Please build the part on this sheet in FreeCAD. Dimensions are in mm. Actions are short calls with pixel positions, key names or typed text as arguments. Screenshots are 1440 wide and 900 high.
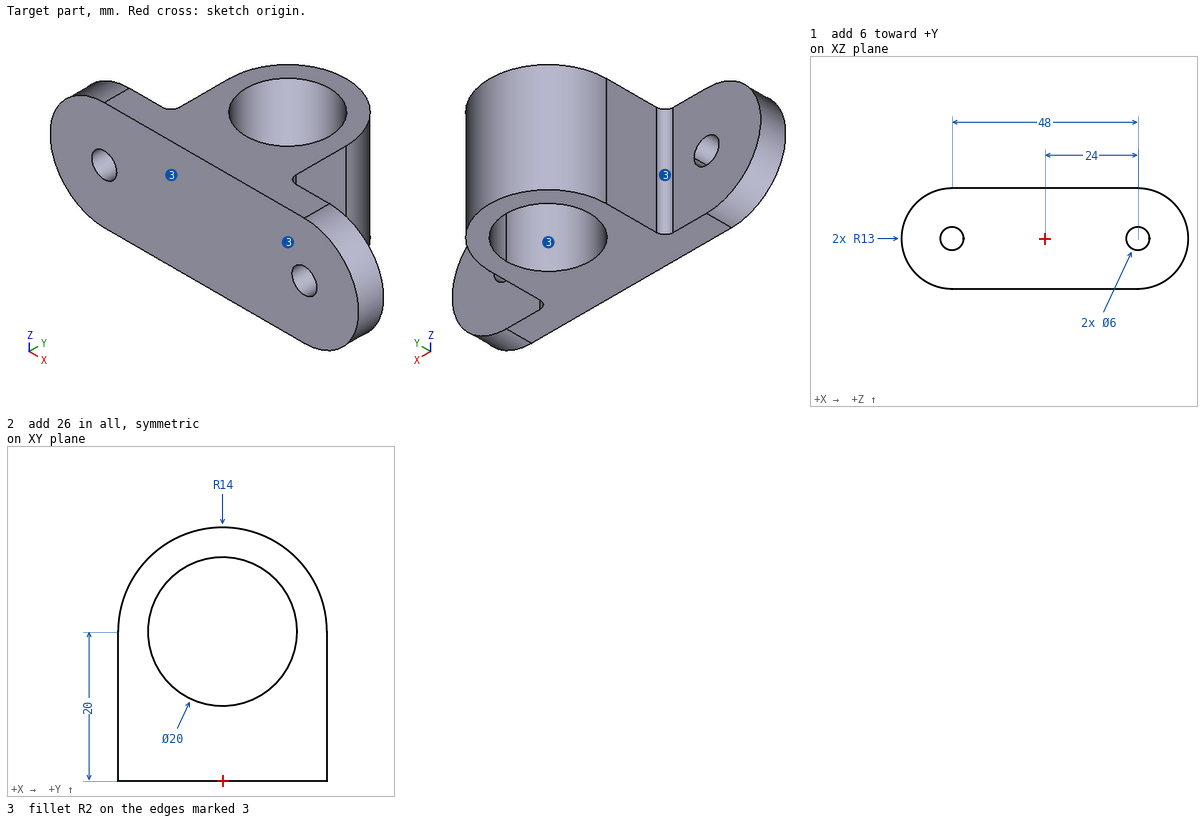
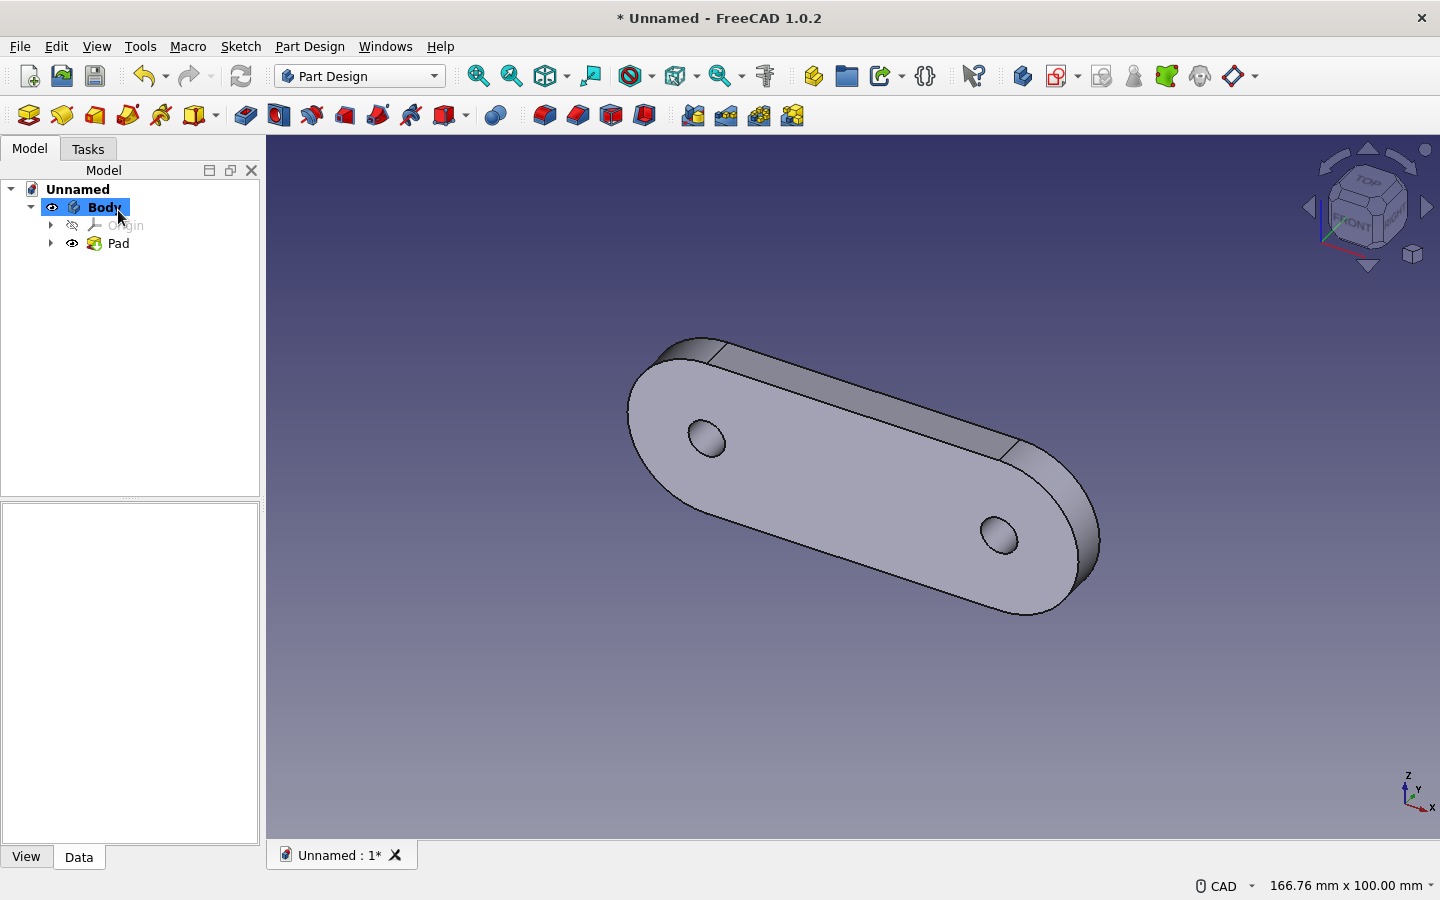
click(1056, 76)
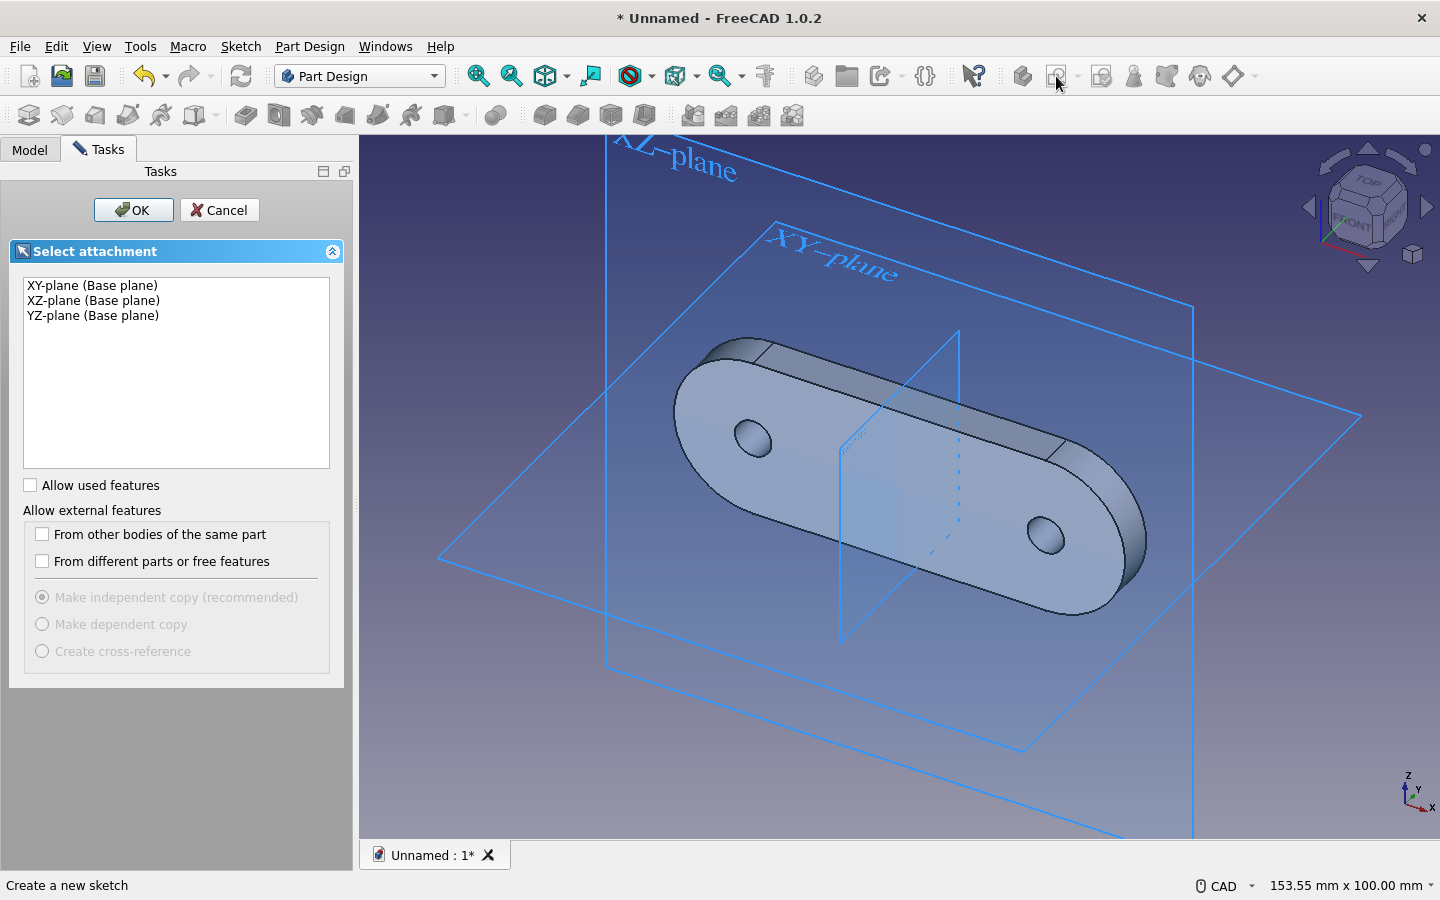
click(84, 286)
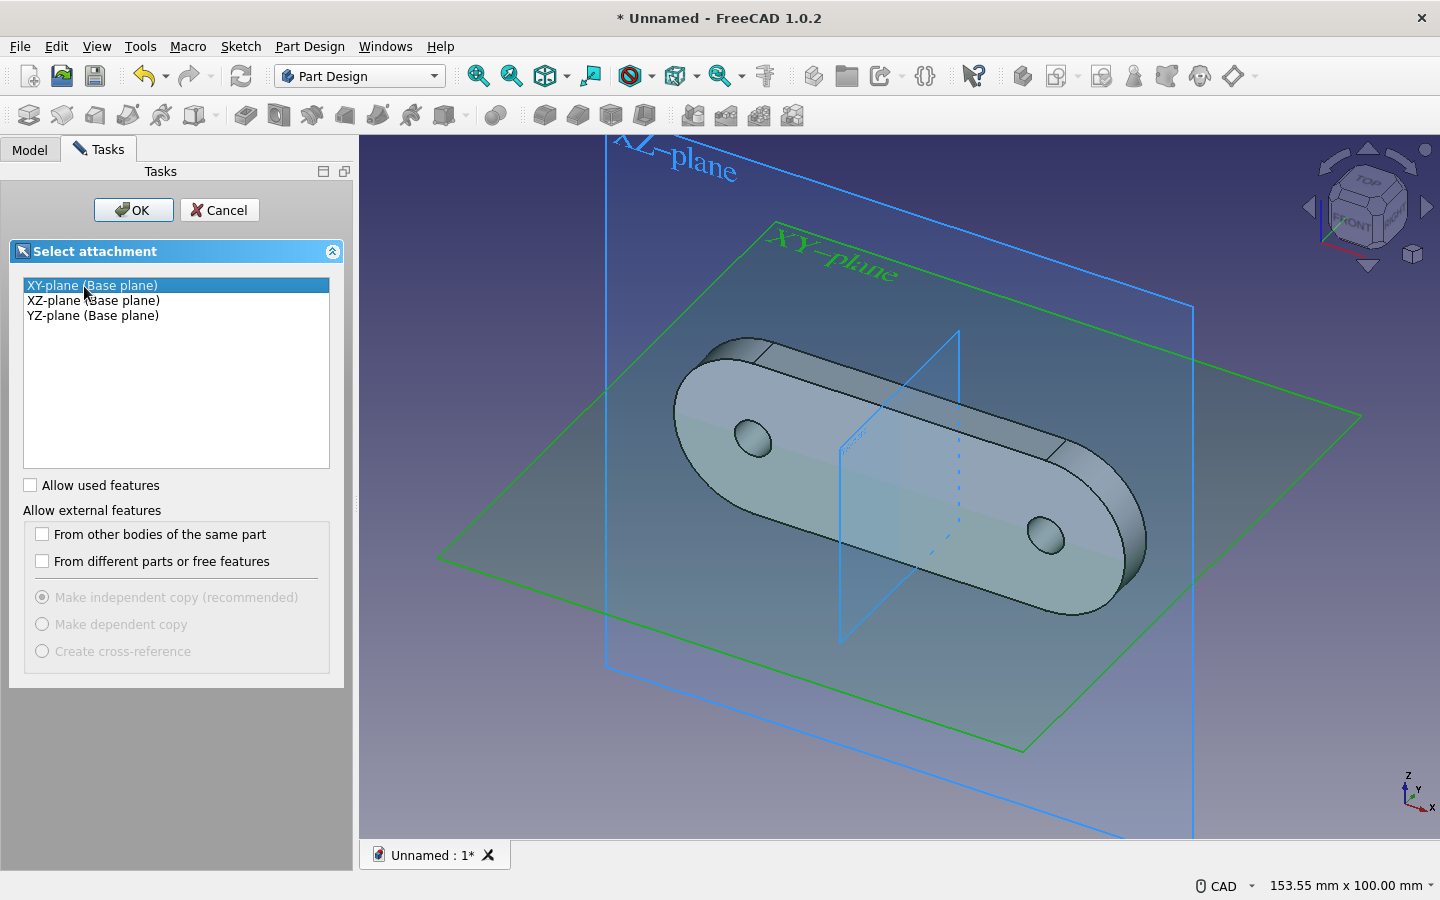
click(134, 210)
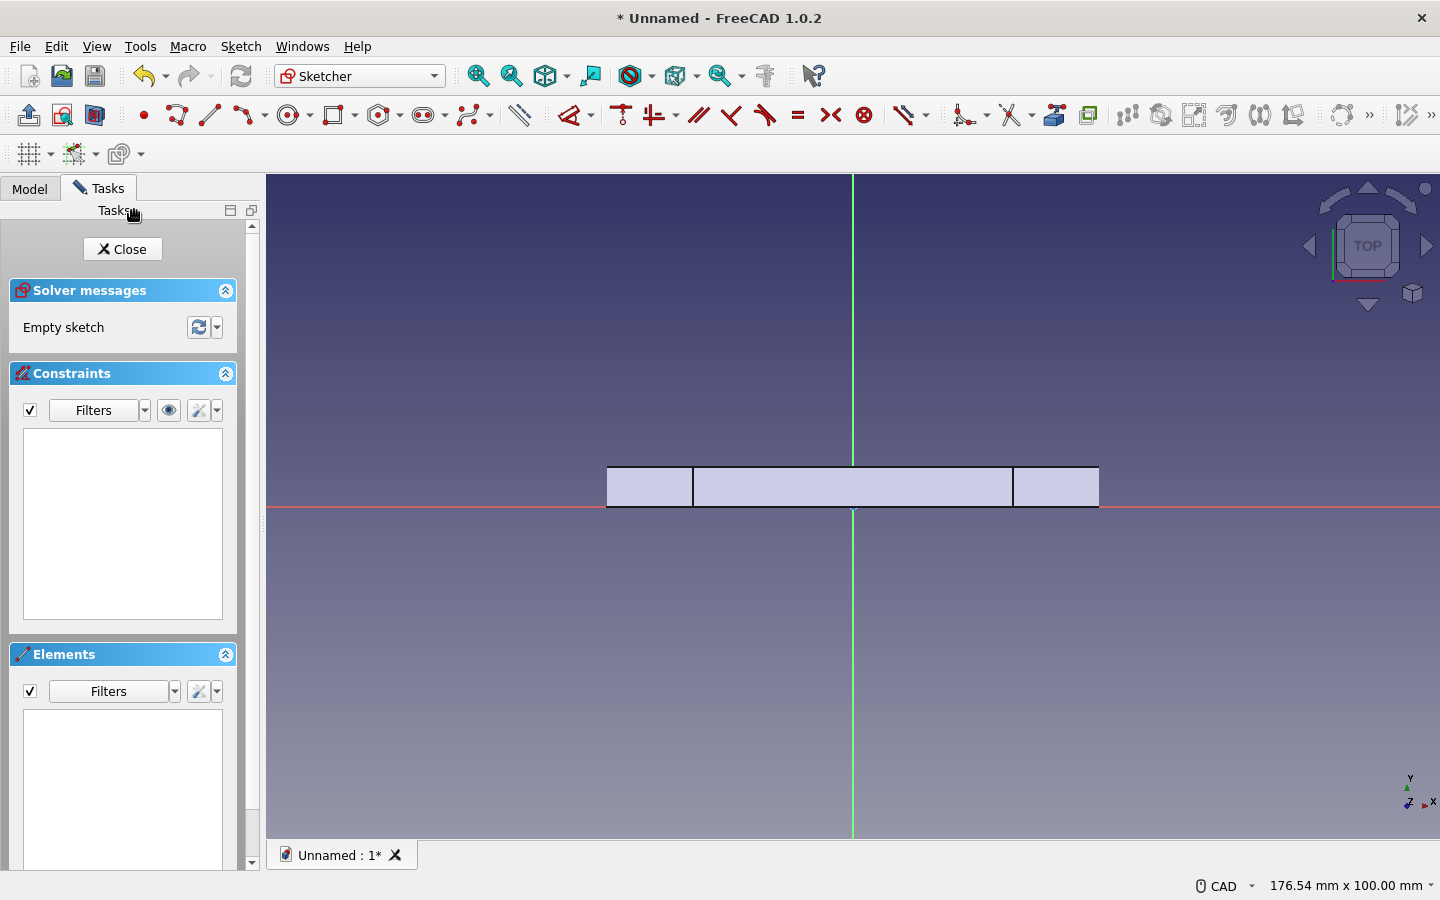
key(q)
key(s)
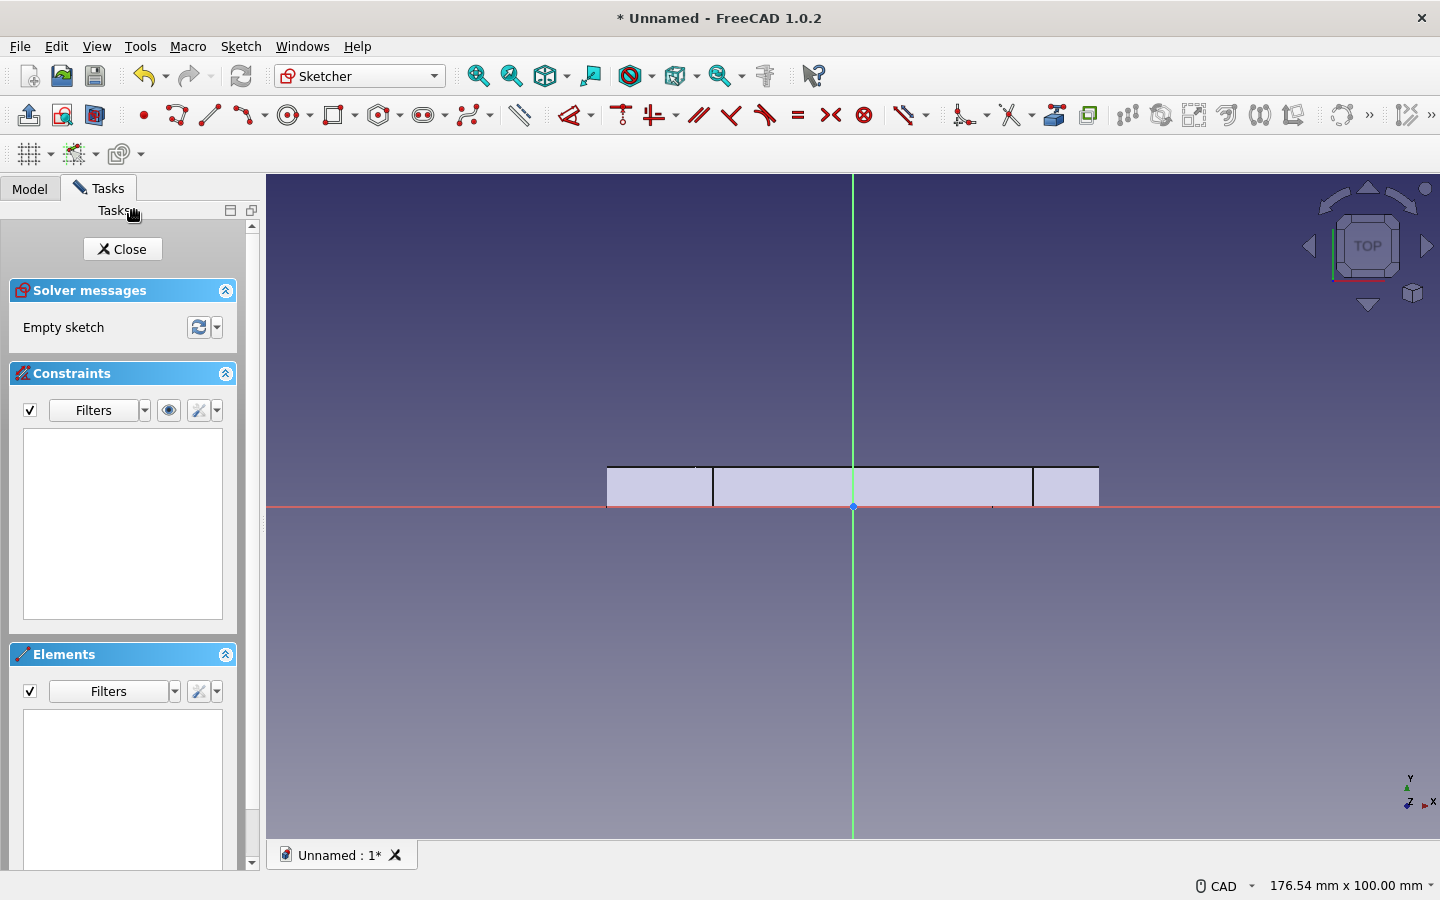
scroll(936, 256, up, 3)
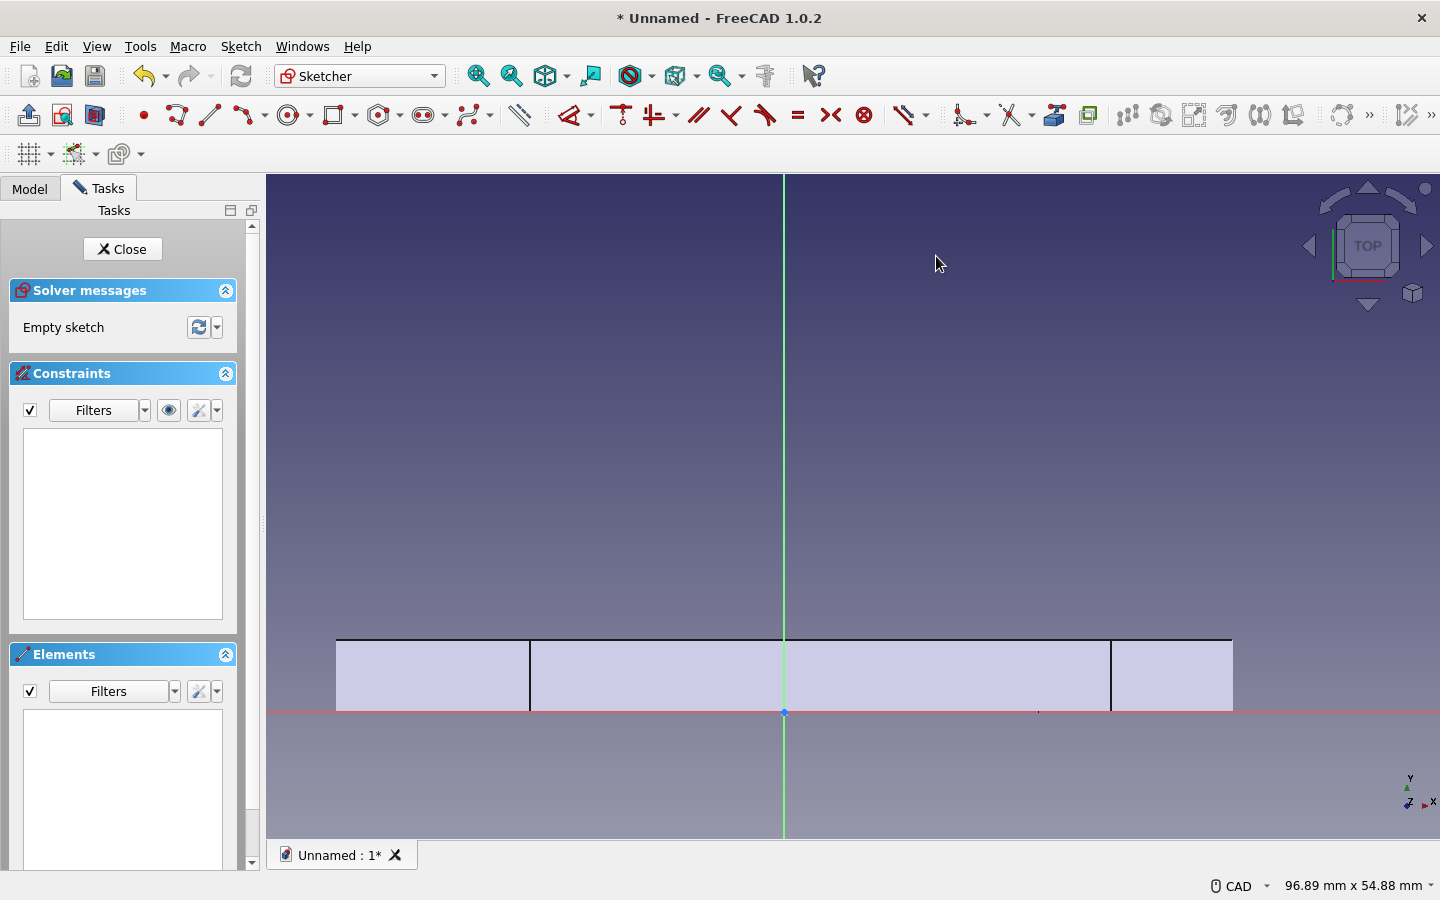
key(g)
key(m)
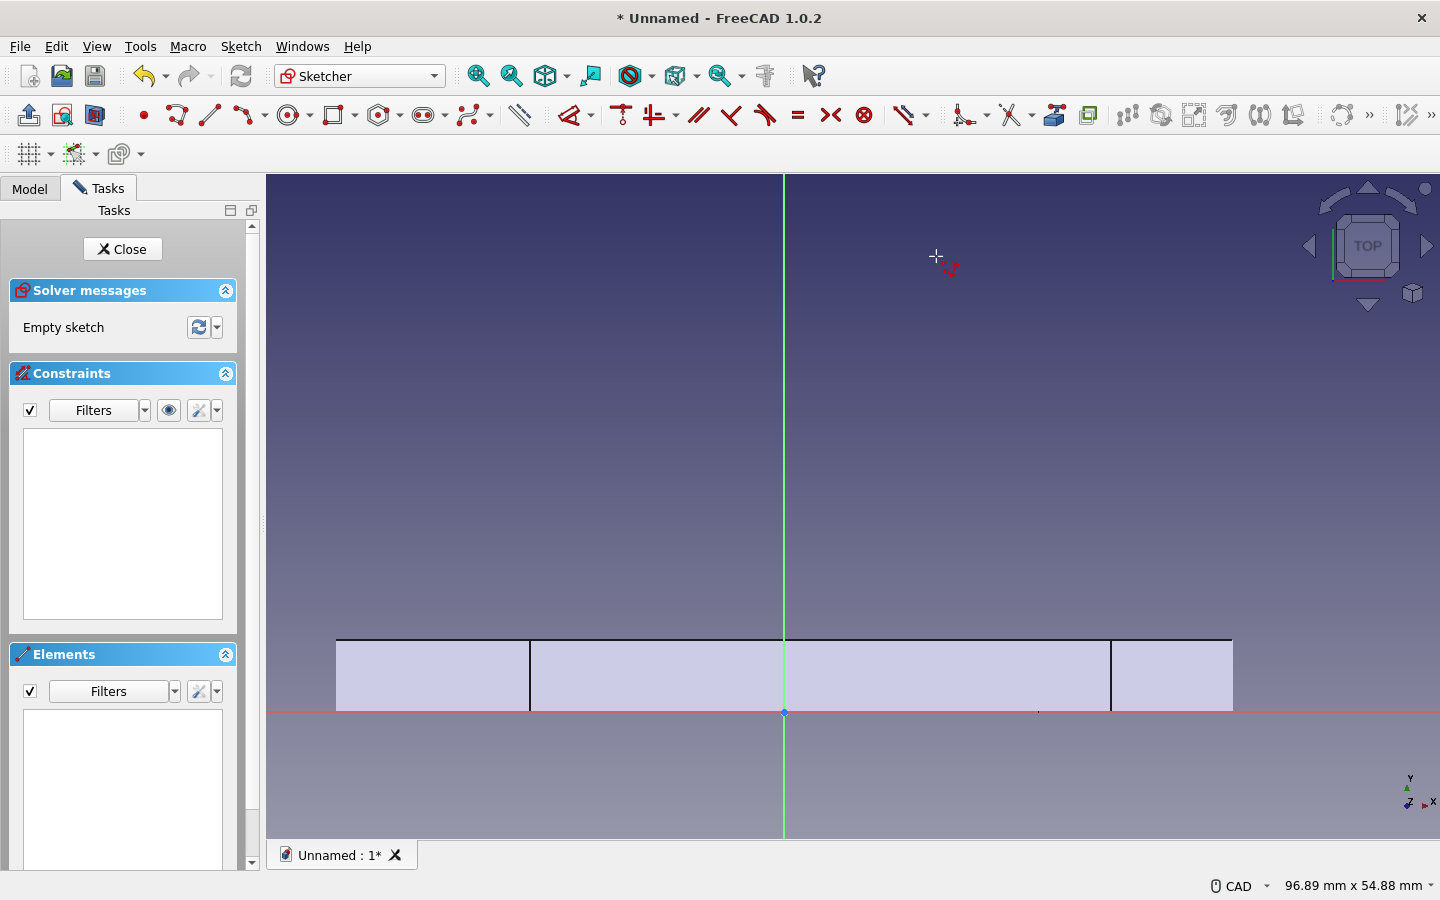
click(615, 470)
click(615, 712)
click(954, 703)
click(954, 470)
right_click(954, 470)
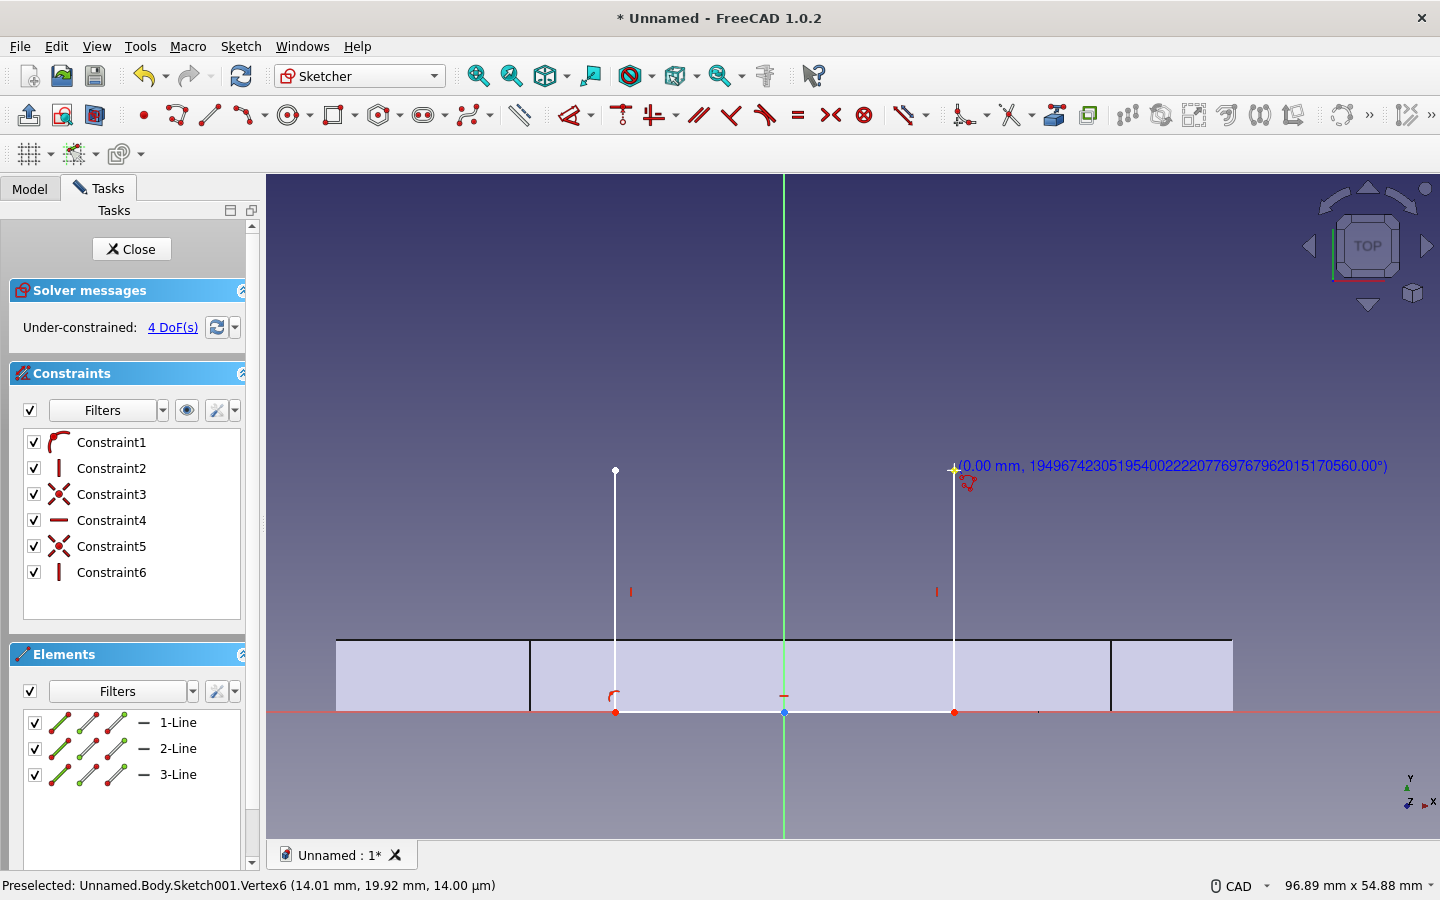
key(g)
key(3)
key(a)